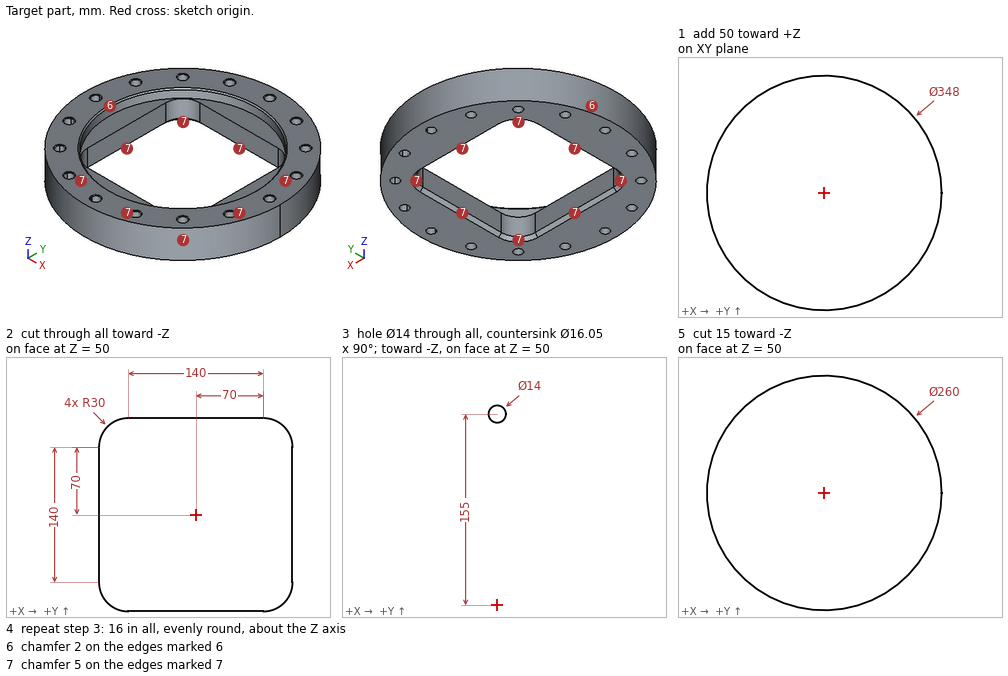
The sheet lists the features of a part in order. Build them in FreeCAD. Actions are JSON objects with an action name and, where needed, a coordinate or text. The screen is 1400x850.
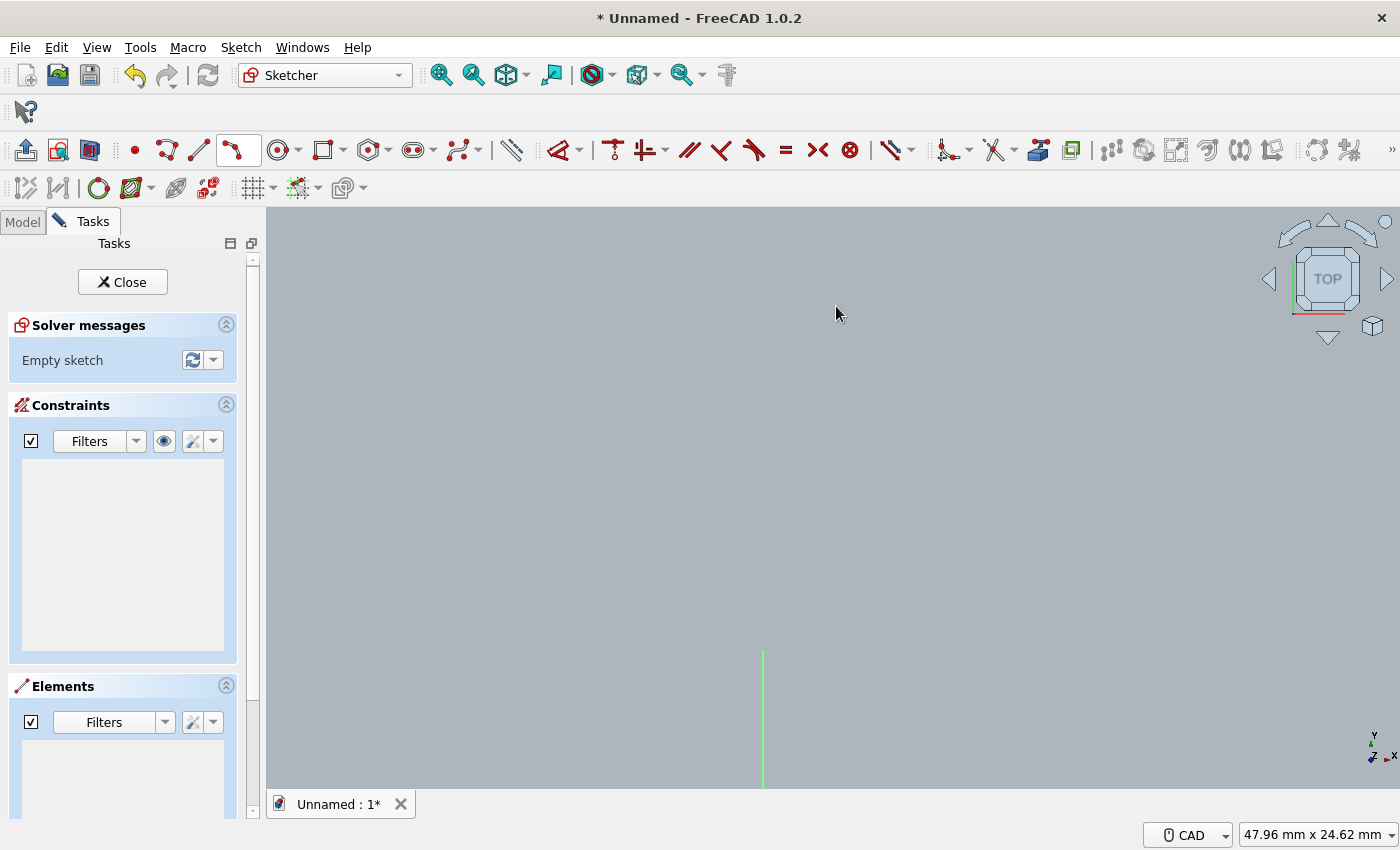
{"action": "left_click", "coordinate": [278, 150]}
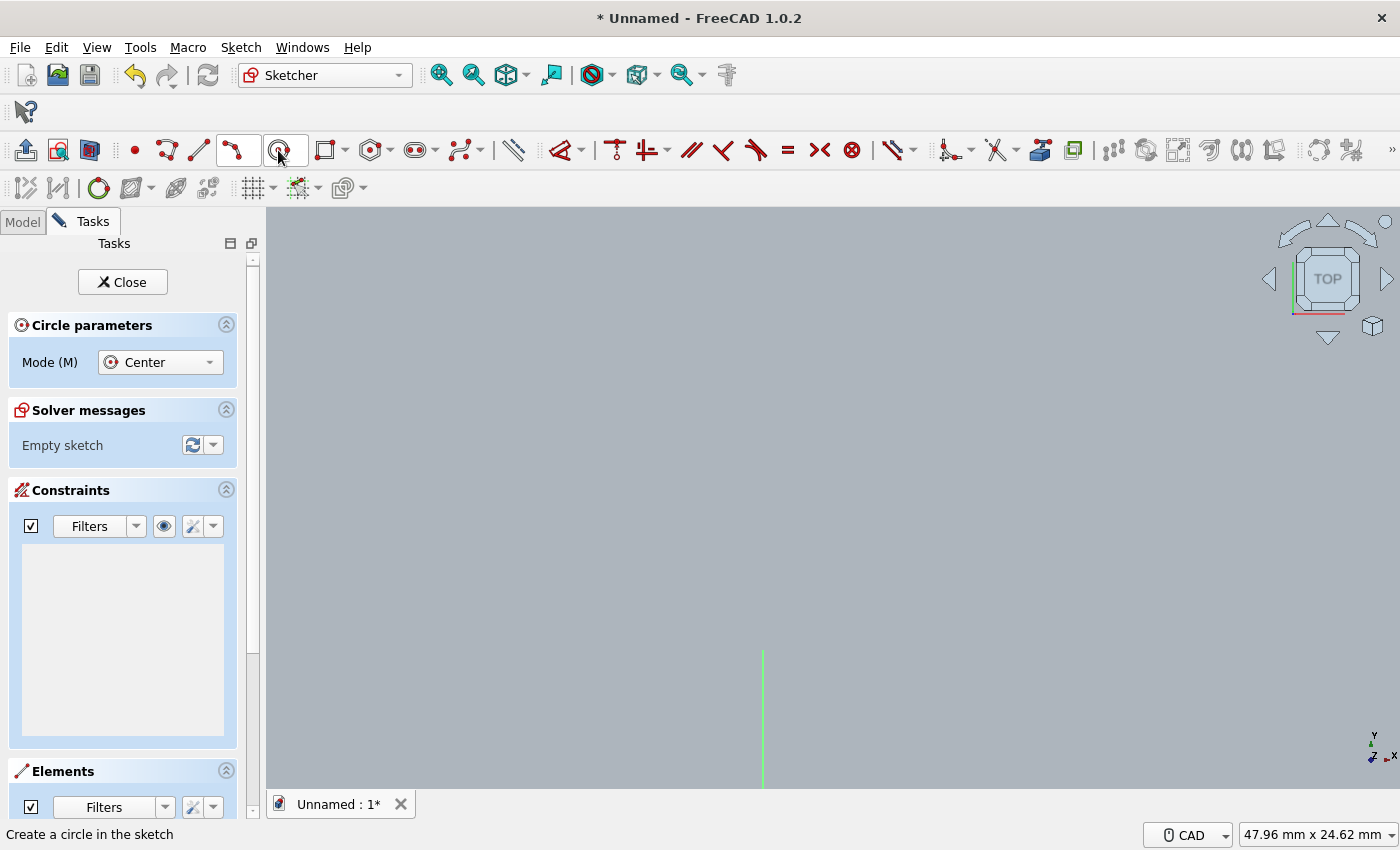
{"action": "left_click", "coordinate": [763, 494]}
{"action": "left_click", "coordinate": [880, 377]}
{"action": "key", "text": "Escape"}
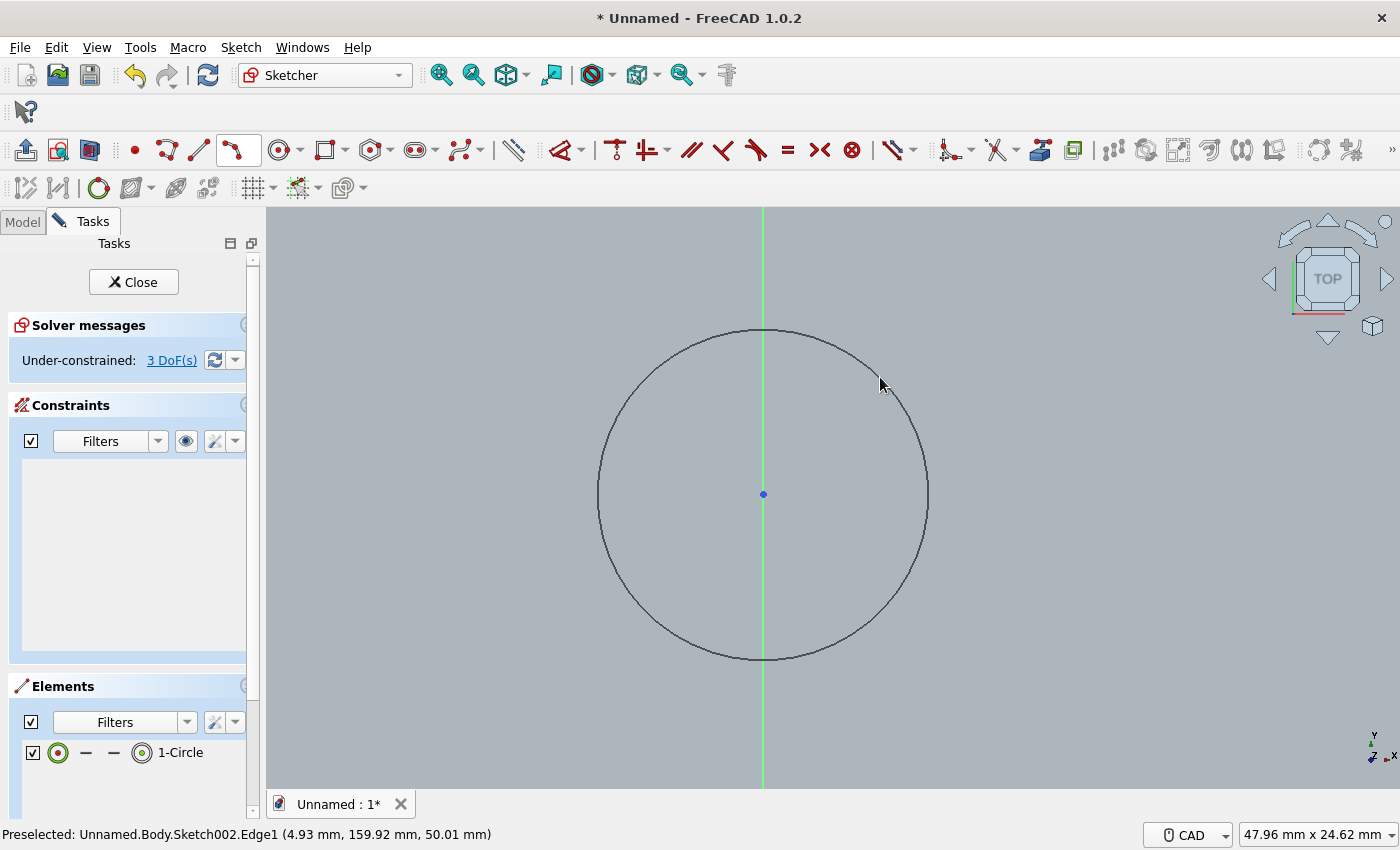
{"action": "left_click", "coordinate": [763, 495]}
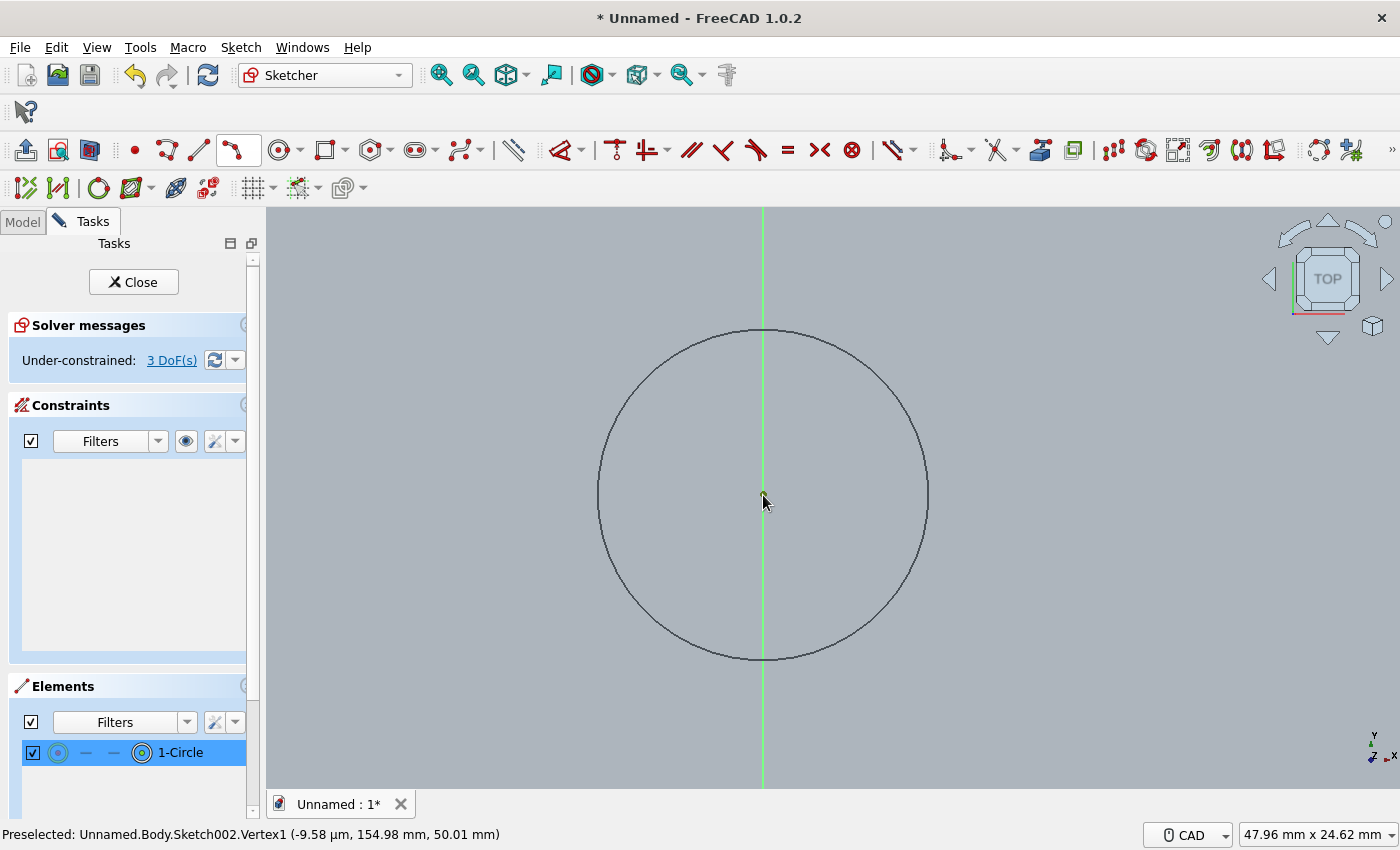
{"action": "left_click", "coordinate": [763, 723]}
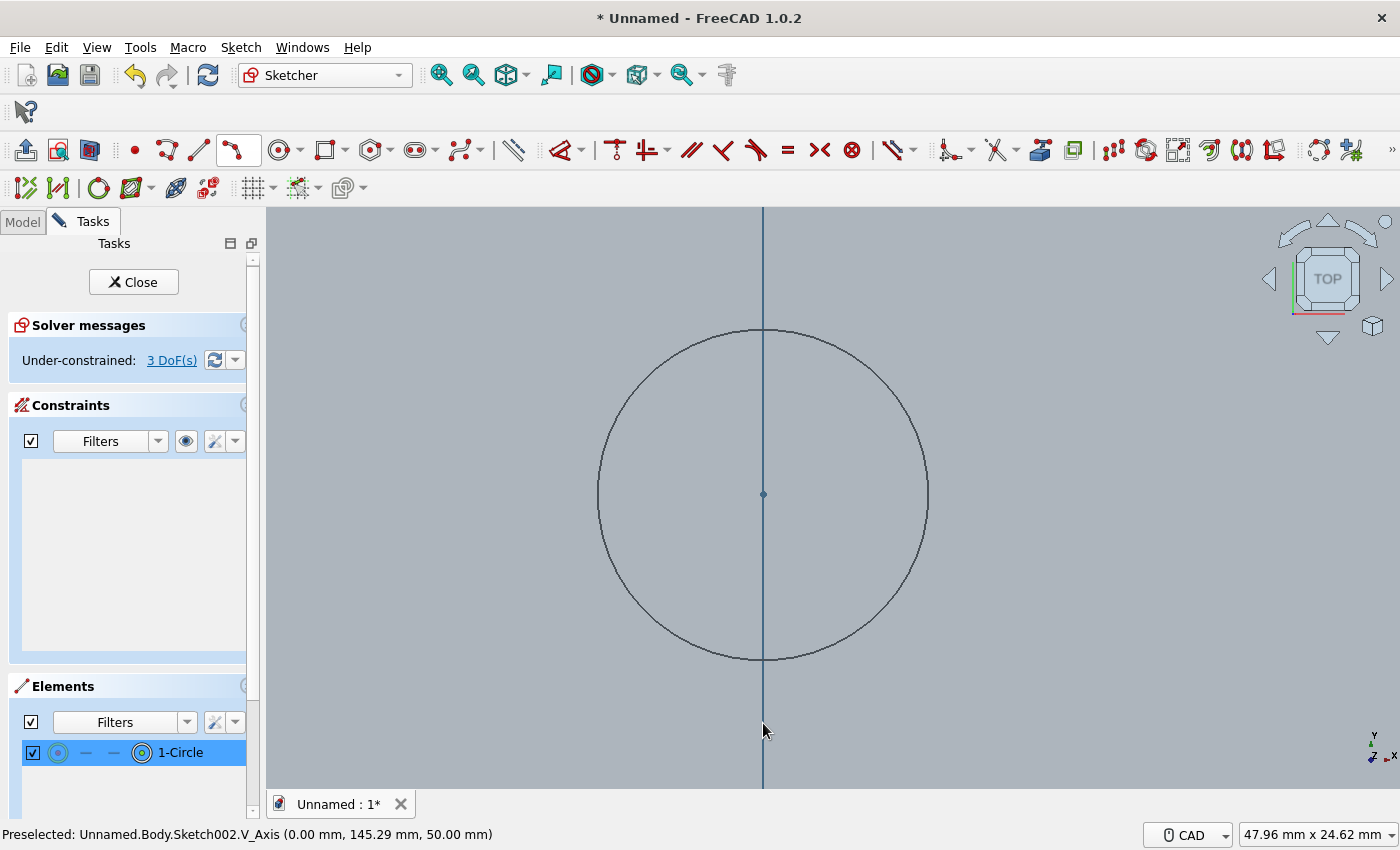
{"action": "left_click", "coordinate": [616, 150]}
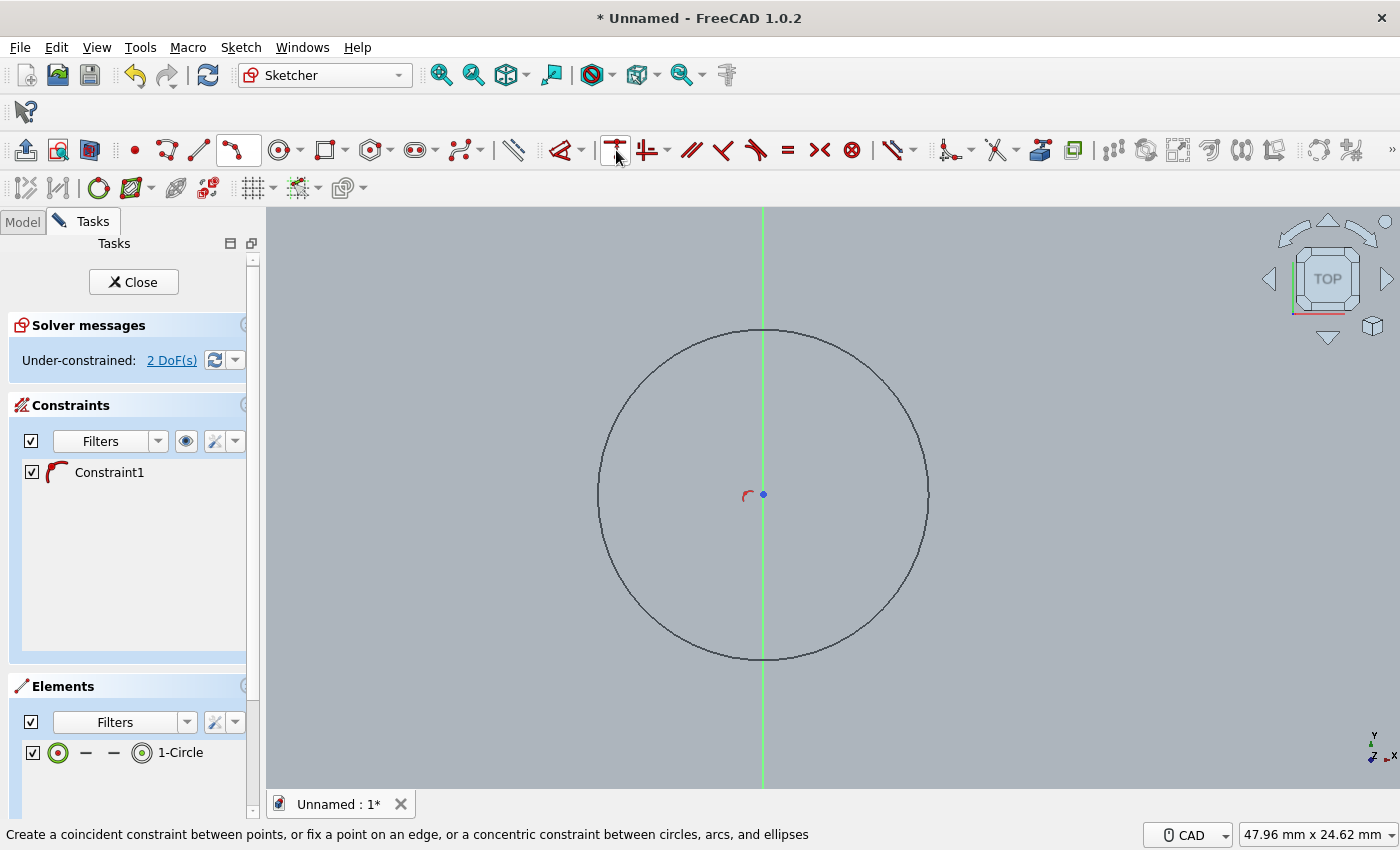
{"action": "left_click", "coordinate": [560, 150]}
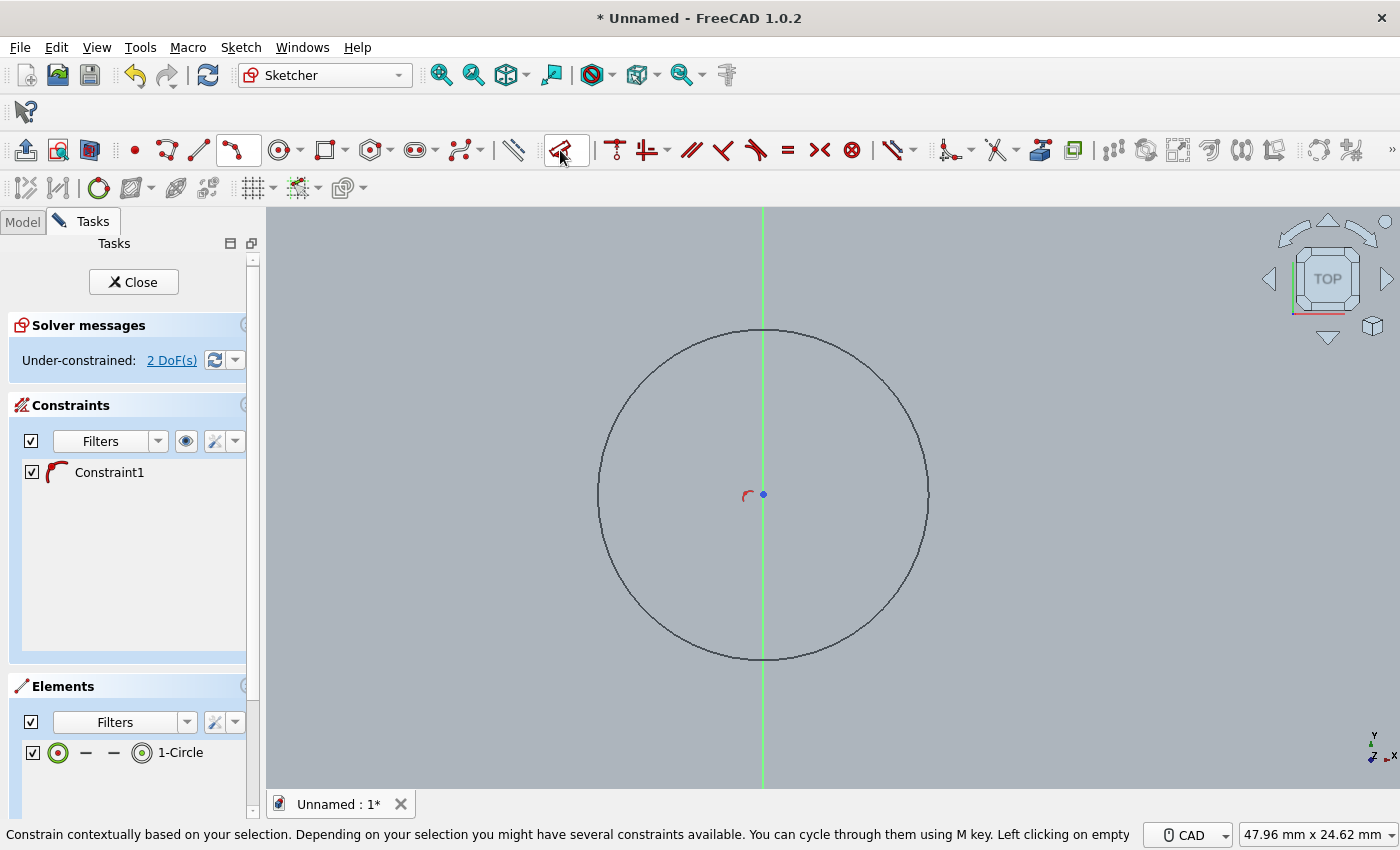
{"action": "left_click", "coordinate": [880, 378]}
{"action": "left_click", "coordinate": [903, 355]}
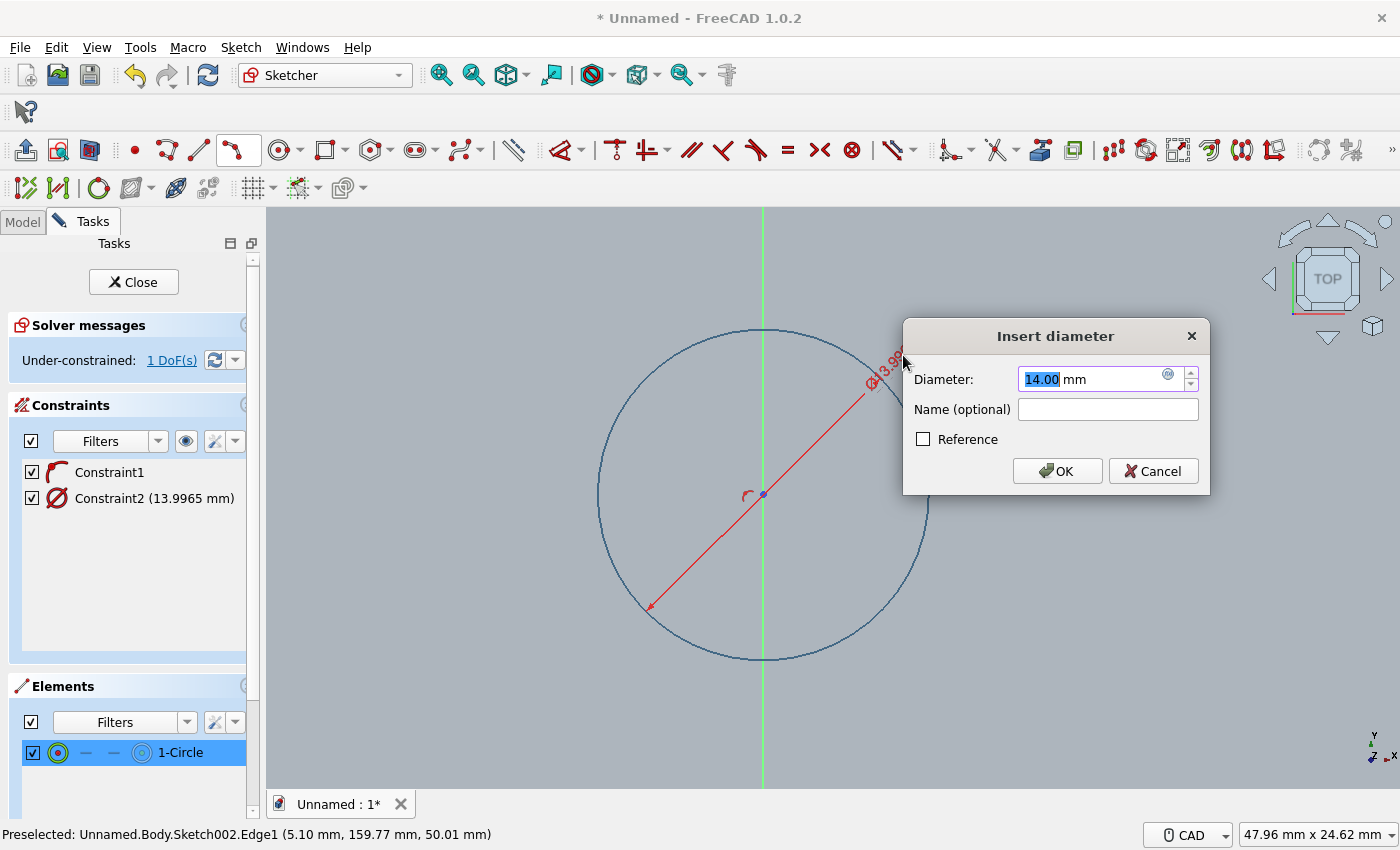
{"action": "type", "text": "14"}
{"action": "key", "text": "Return"}